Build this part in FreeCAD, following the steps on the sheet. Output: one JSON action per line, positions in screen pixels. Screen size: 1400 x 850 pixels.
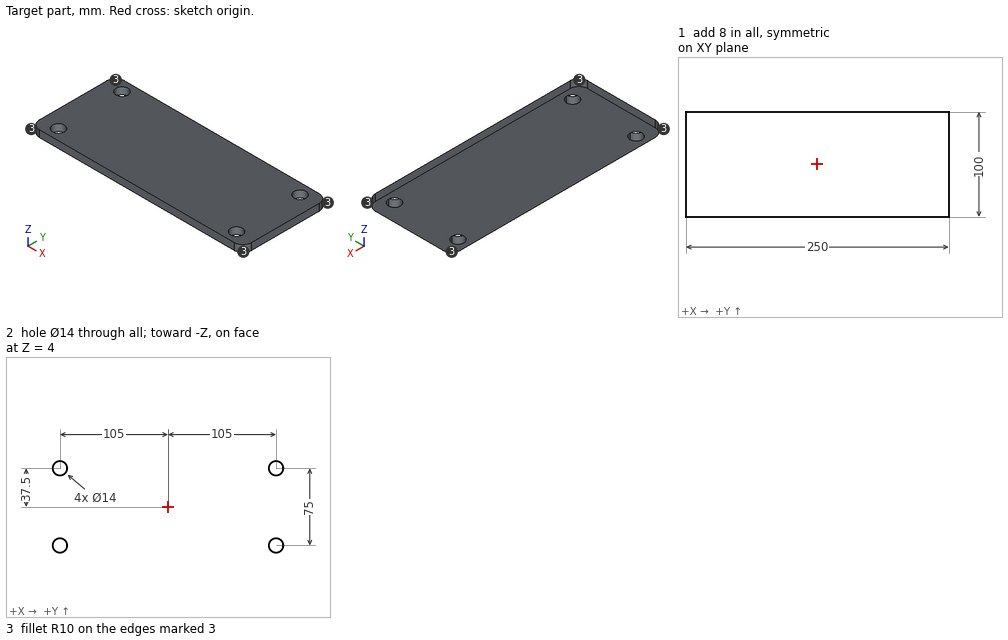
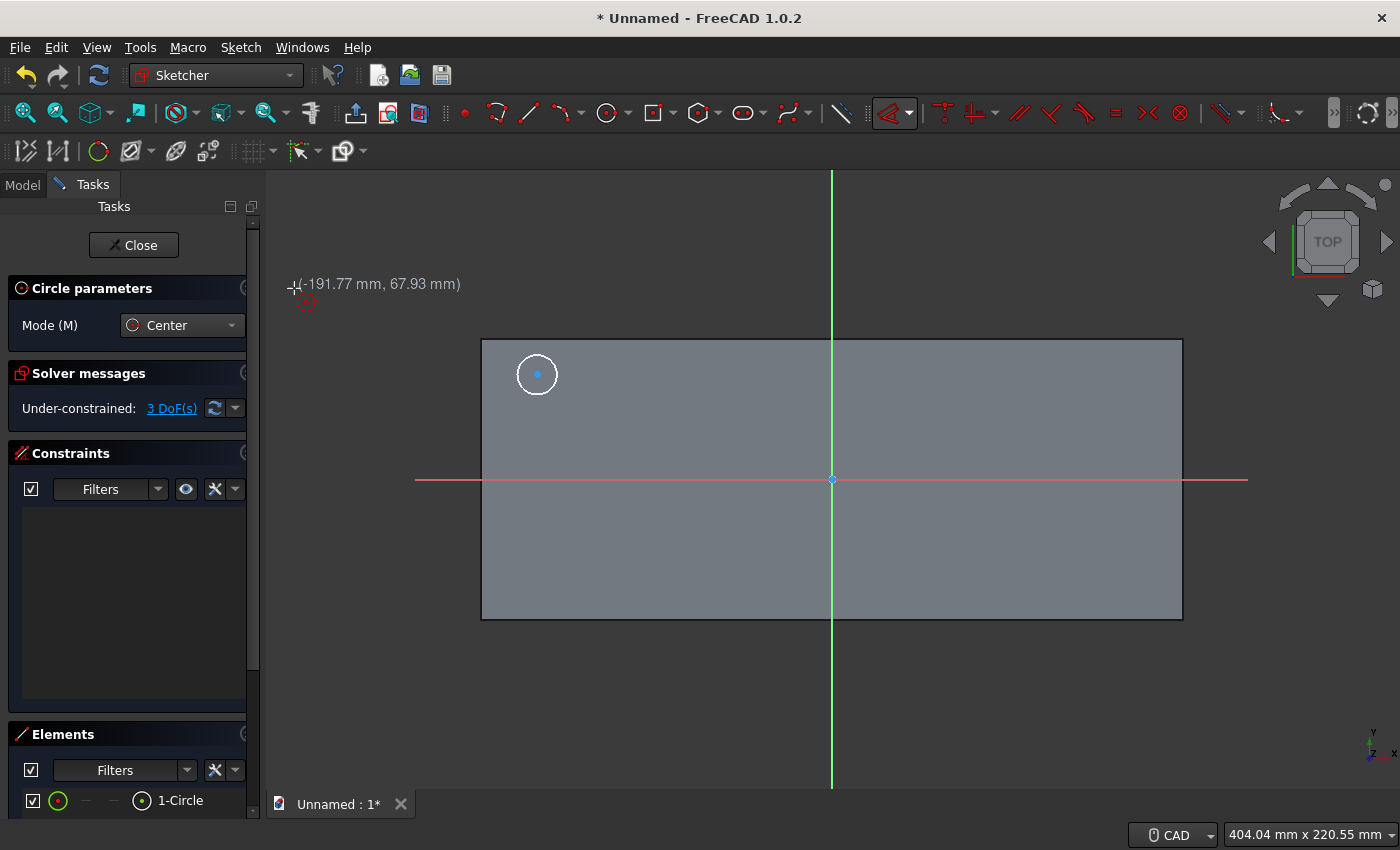
{"action": "left_click", "coordinate": [1127, 374]}
{"action": "left_click", "coordinate": [1141, 360]}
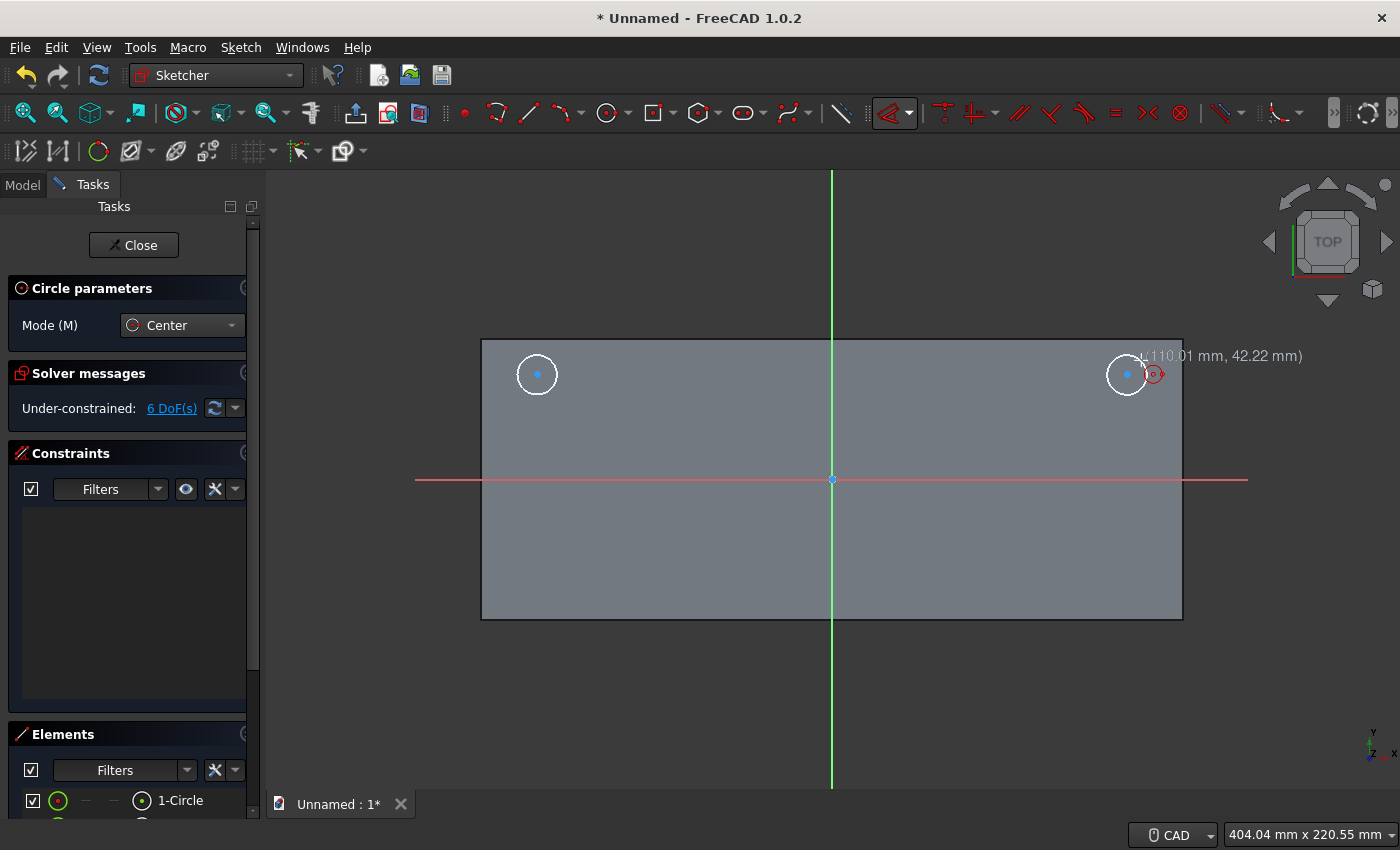
{"action": "left_click", "coordinate": [1127, 585]}
{"action": "left_click", "coordinate": [1141, 571]}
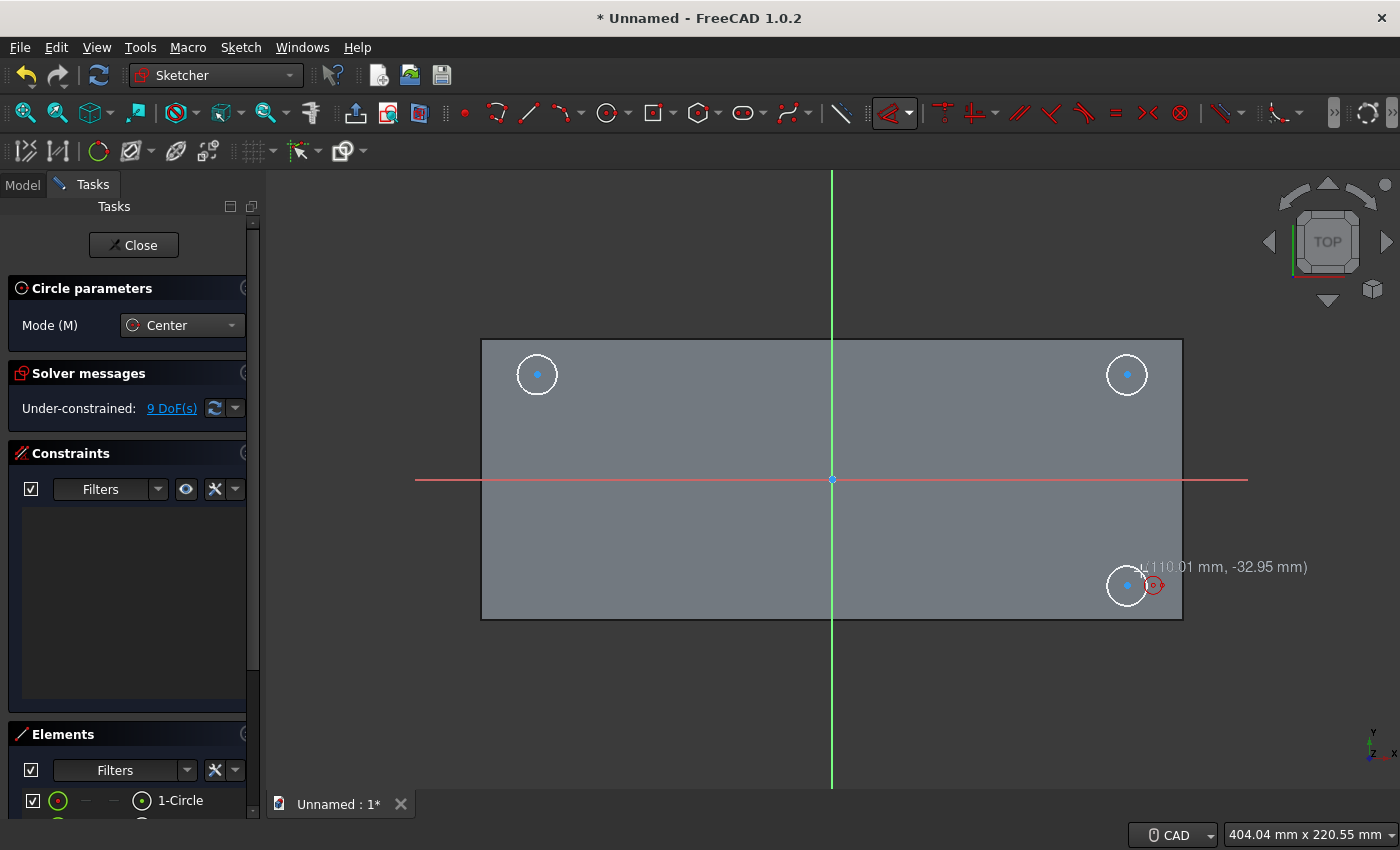
{"action": "left_click", "coordinate": [538, 585]}
{"action": "left_click", "coordinate": [551, 571]}
{"action": "key", "text": "Escape"}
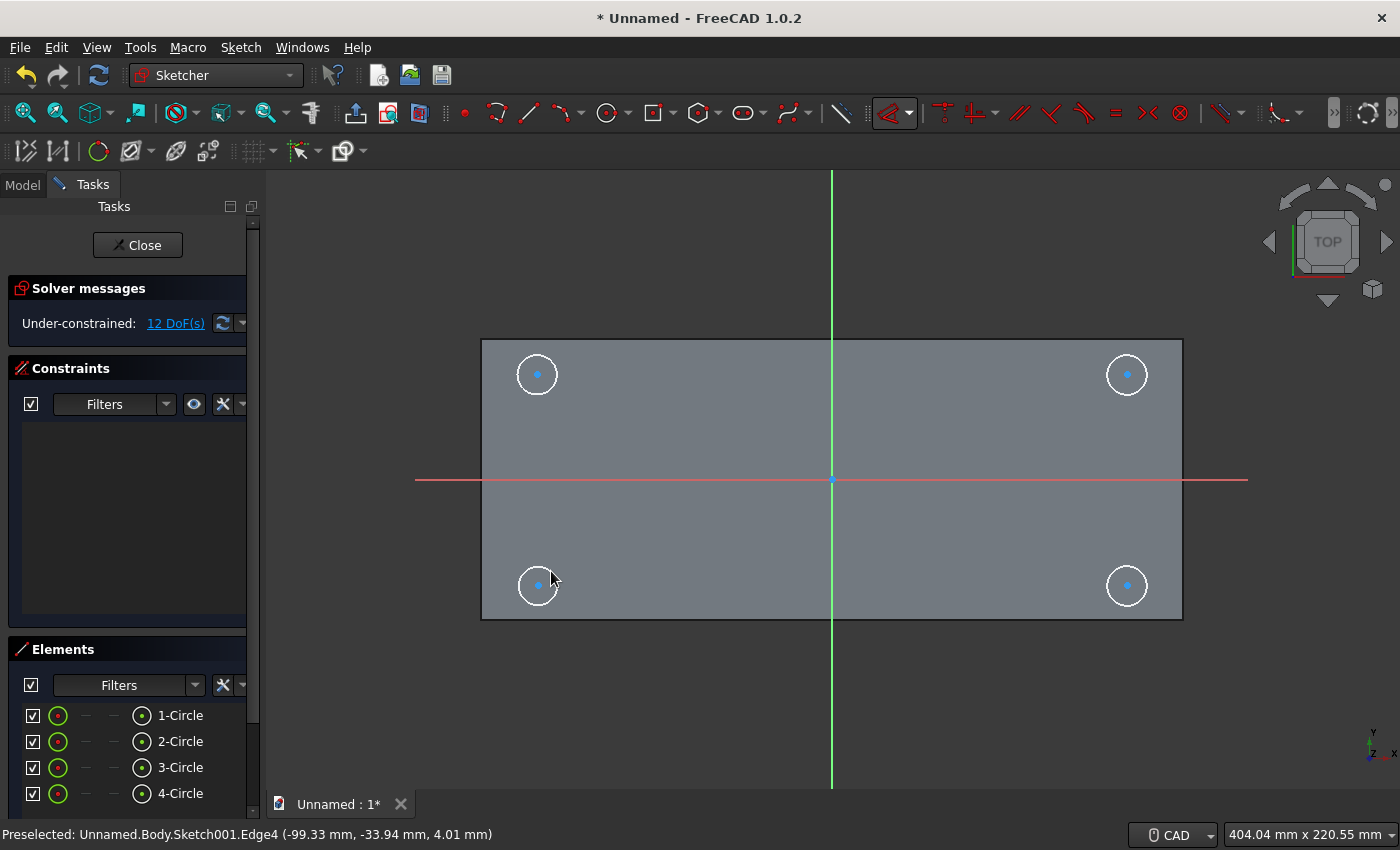
{"action": "left_click", "coordinate": [551, 361]}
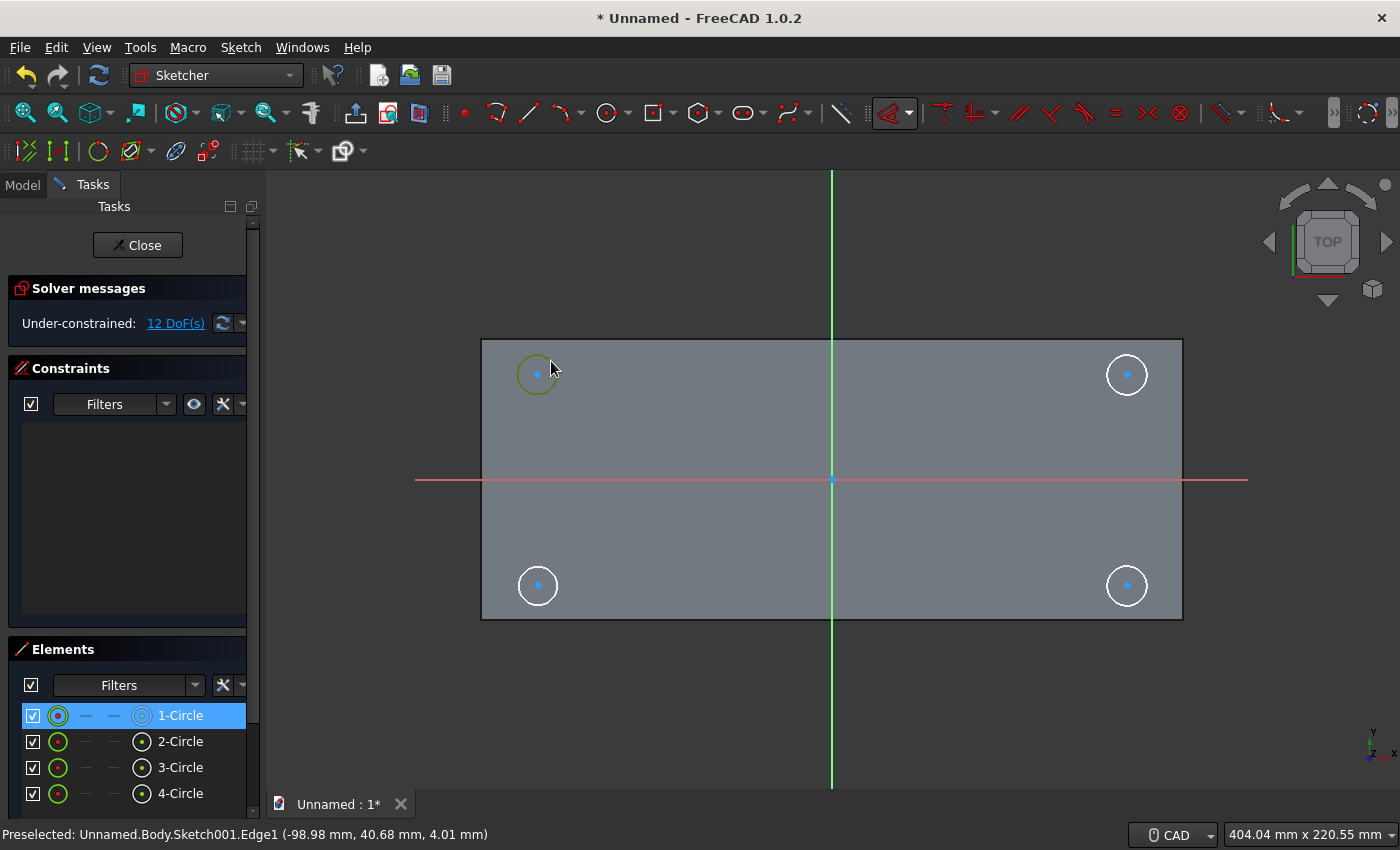
{"action": "left_click", "coordinate": [1141, 361]}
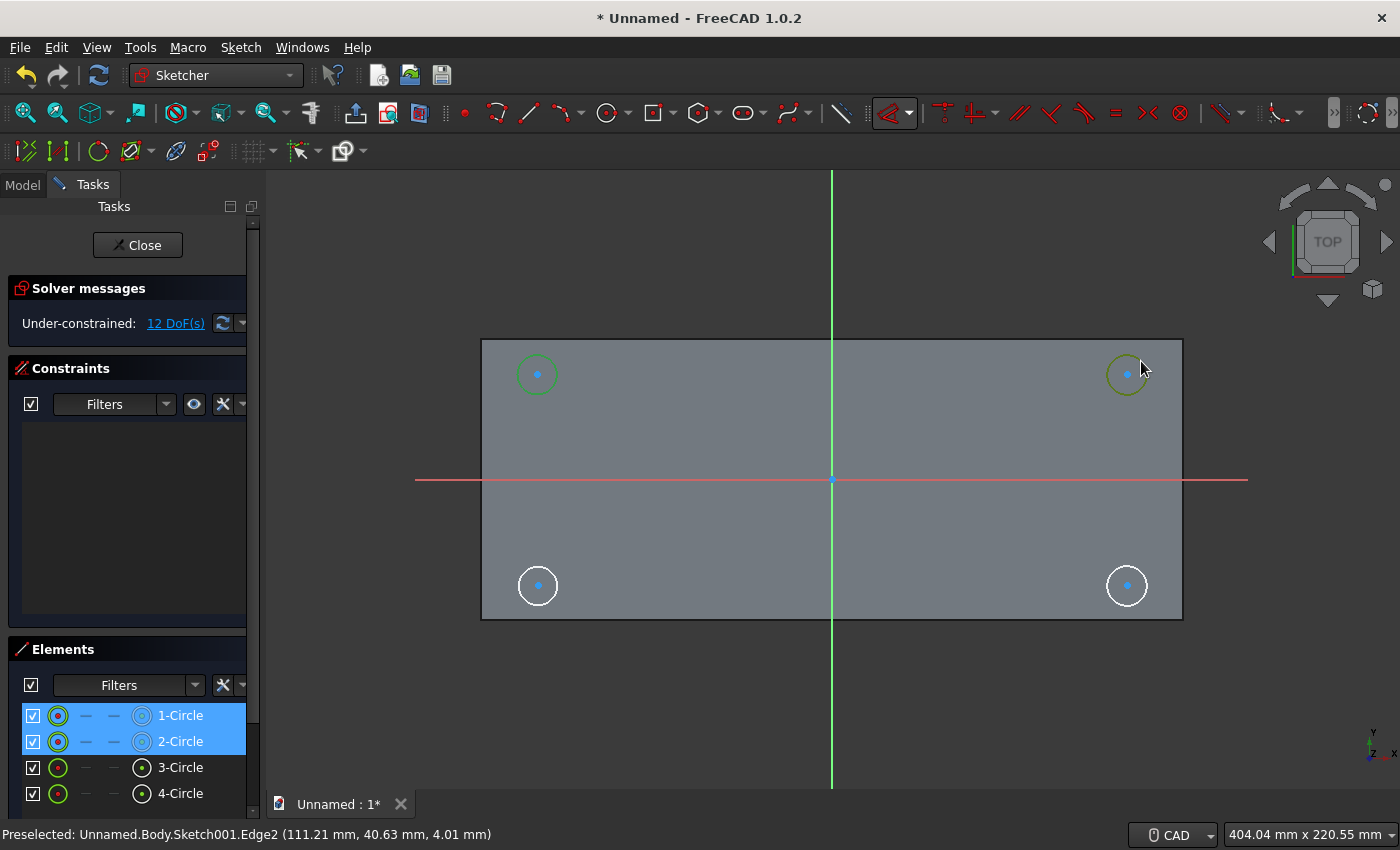
{"action": "left_click", "coordinate": [1141, 572]}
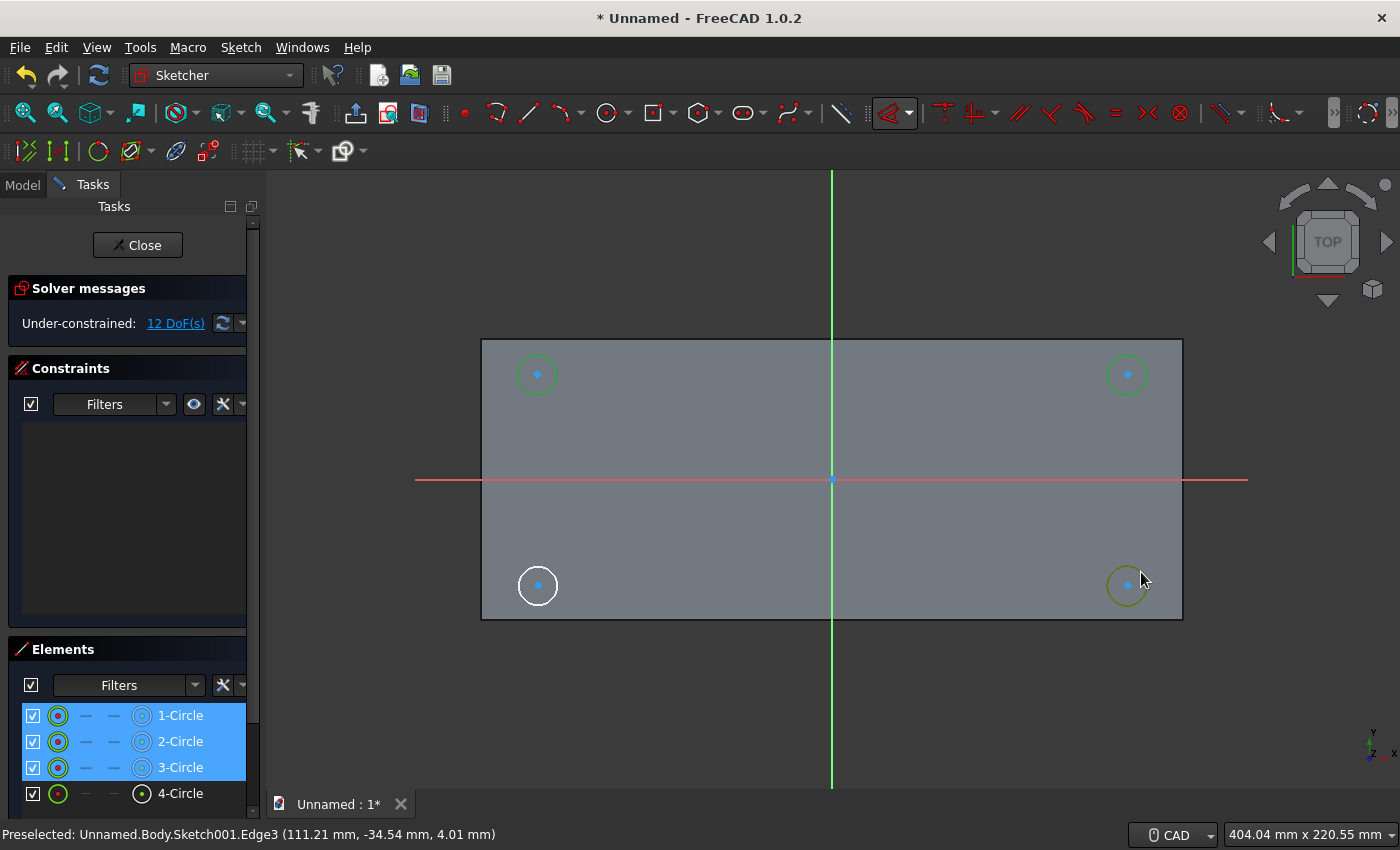
{"action": "left_click", "coordinate": [551, 572]}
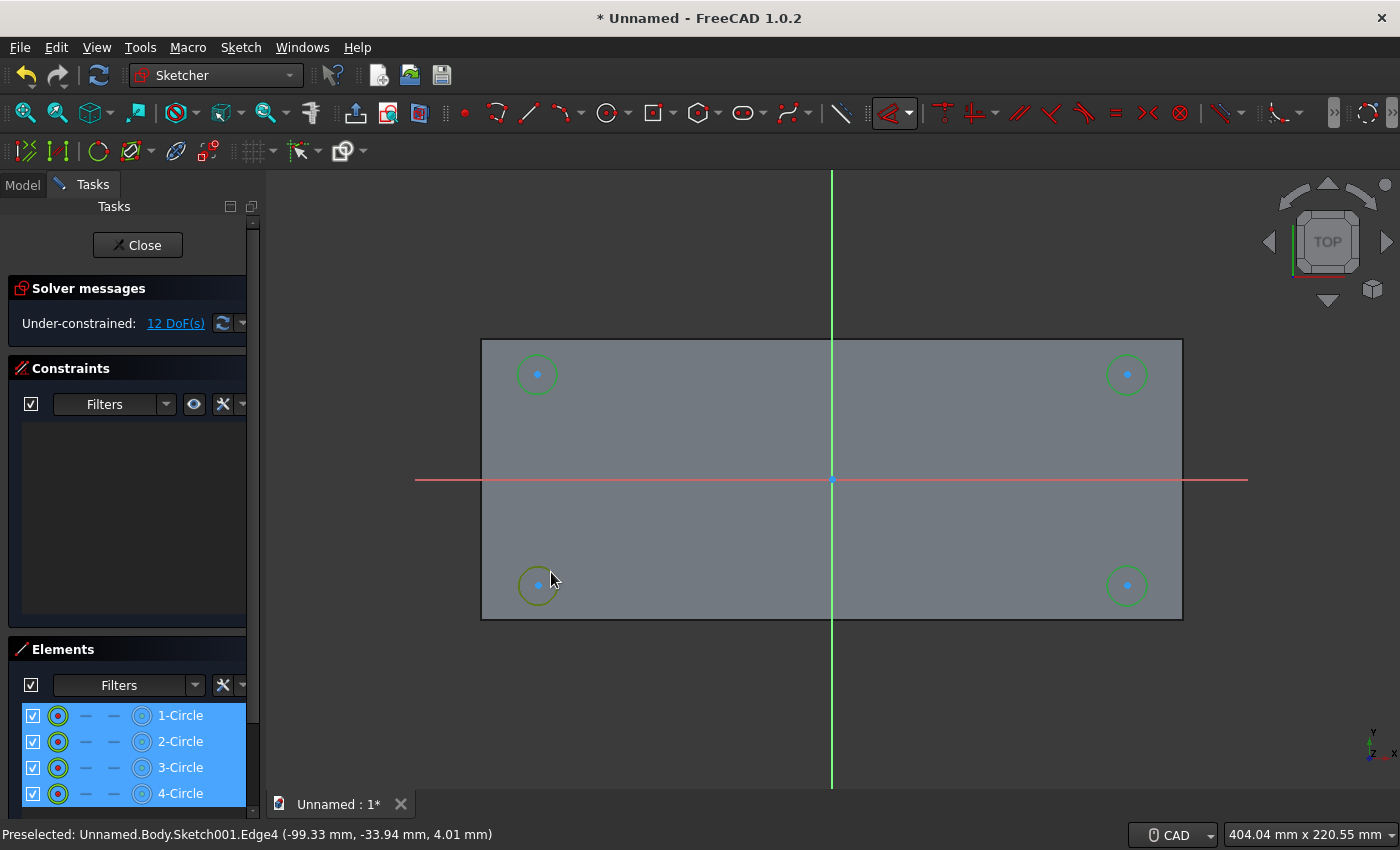
{"action": "left_click", "coordinate": [1116, 114]}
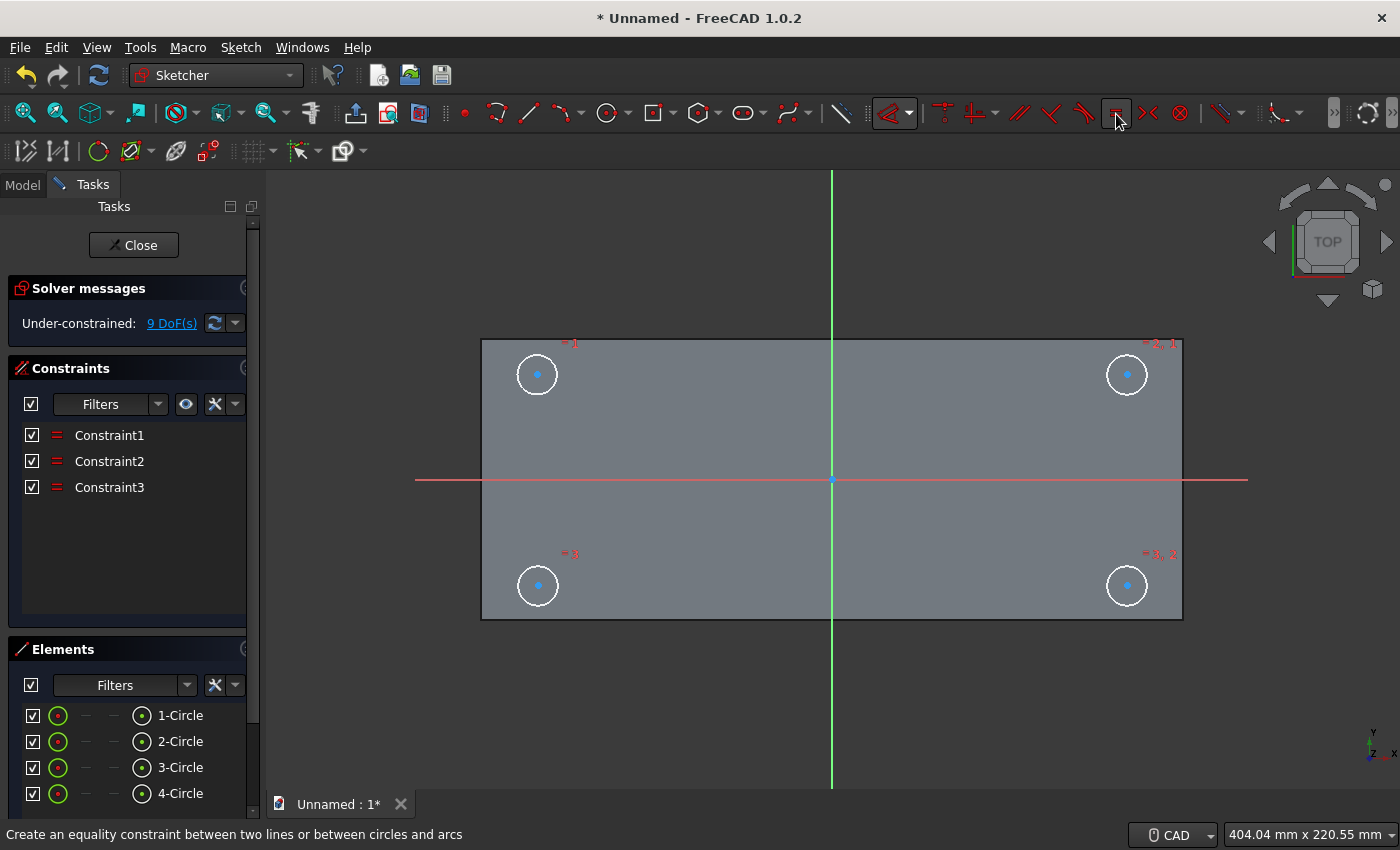
{"action": "left_click", "coordinate": [537, 375]}